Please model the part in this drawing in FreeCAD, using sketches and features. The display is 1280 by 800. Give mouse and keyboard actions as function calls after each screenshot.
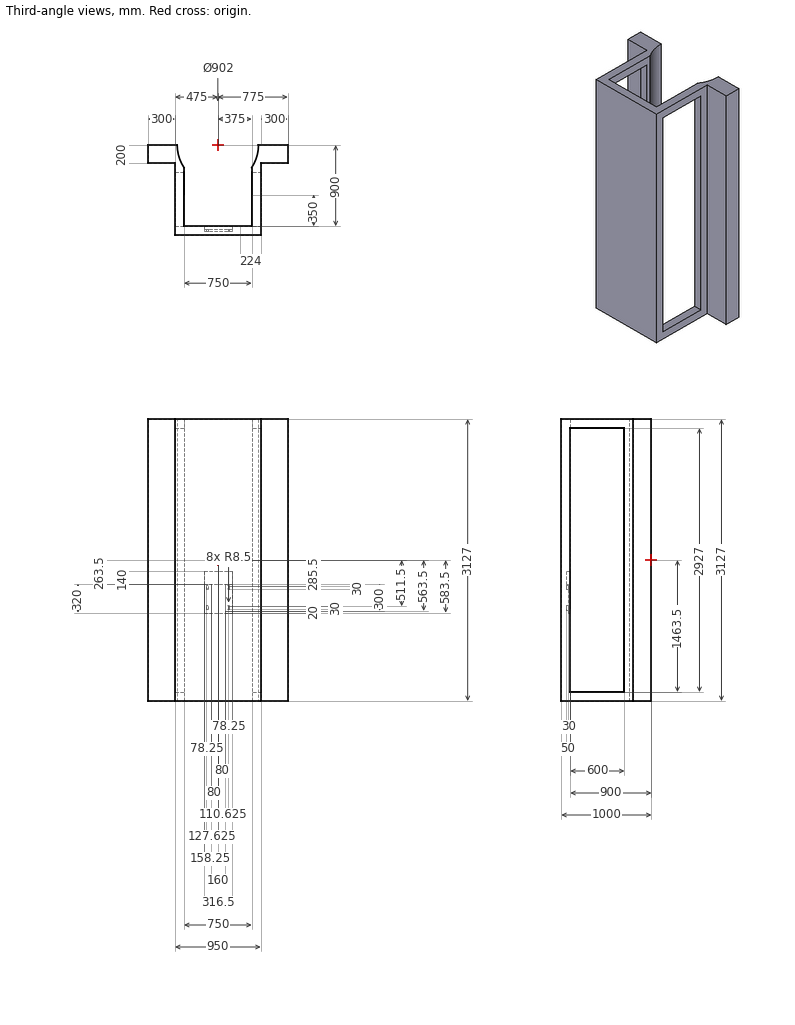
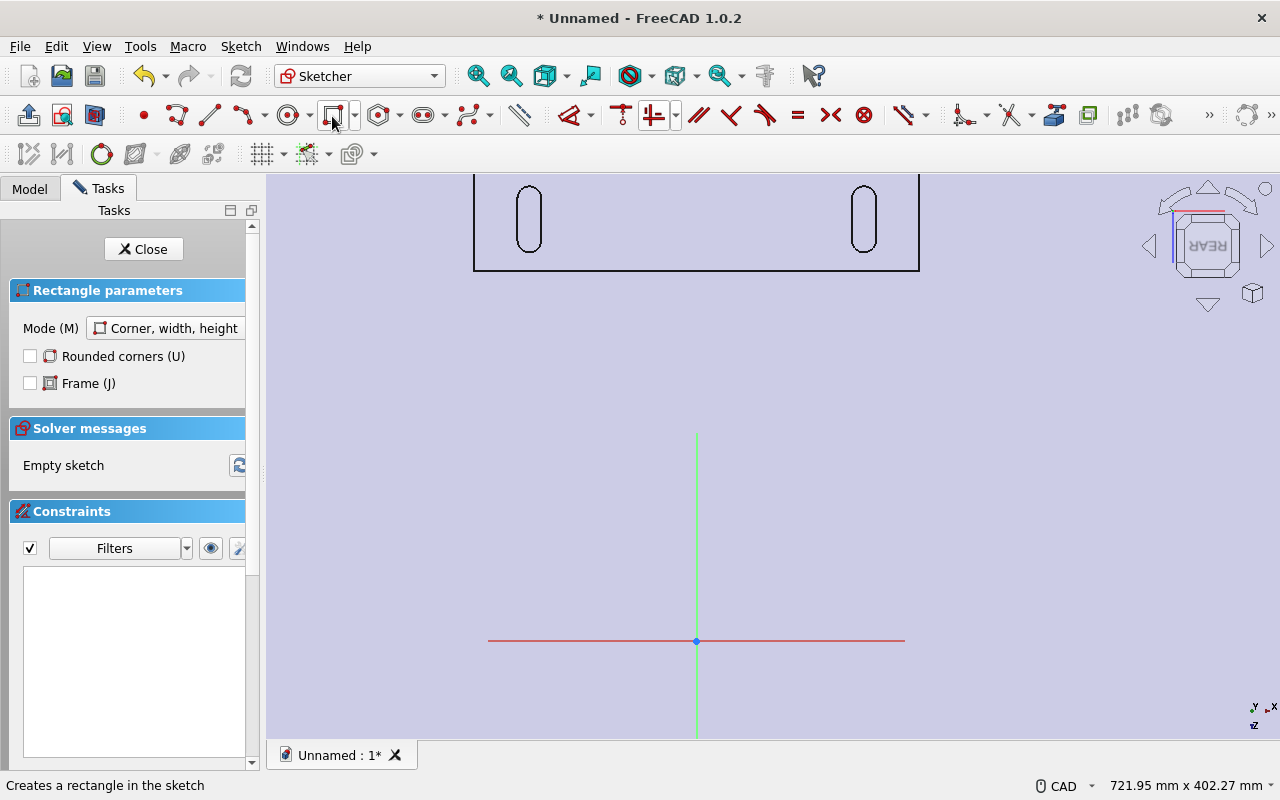
click(474, 271)
click(919, 468)
key(Escape)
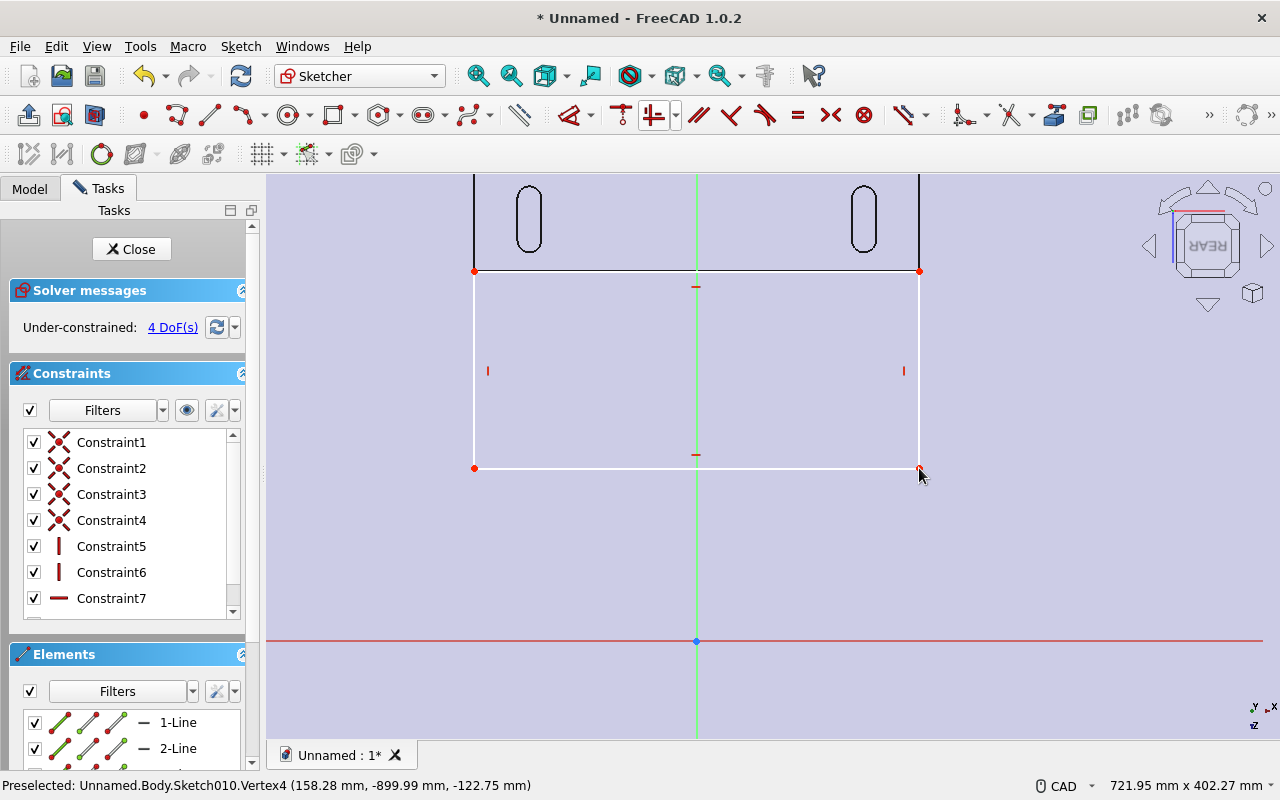
click(568, 116)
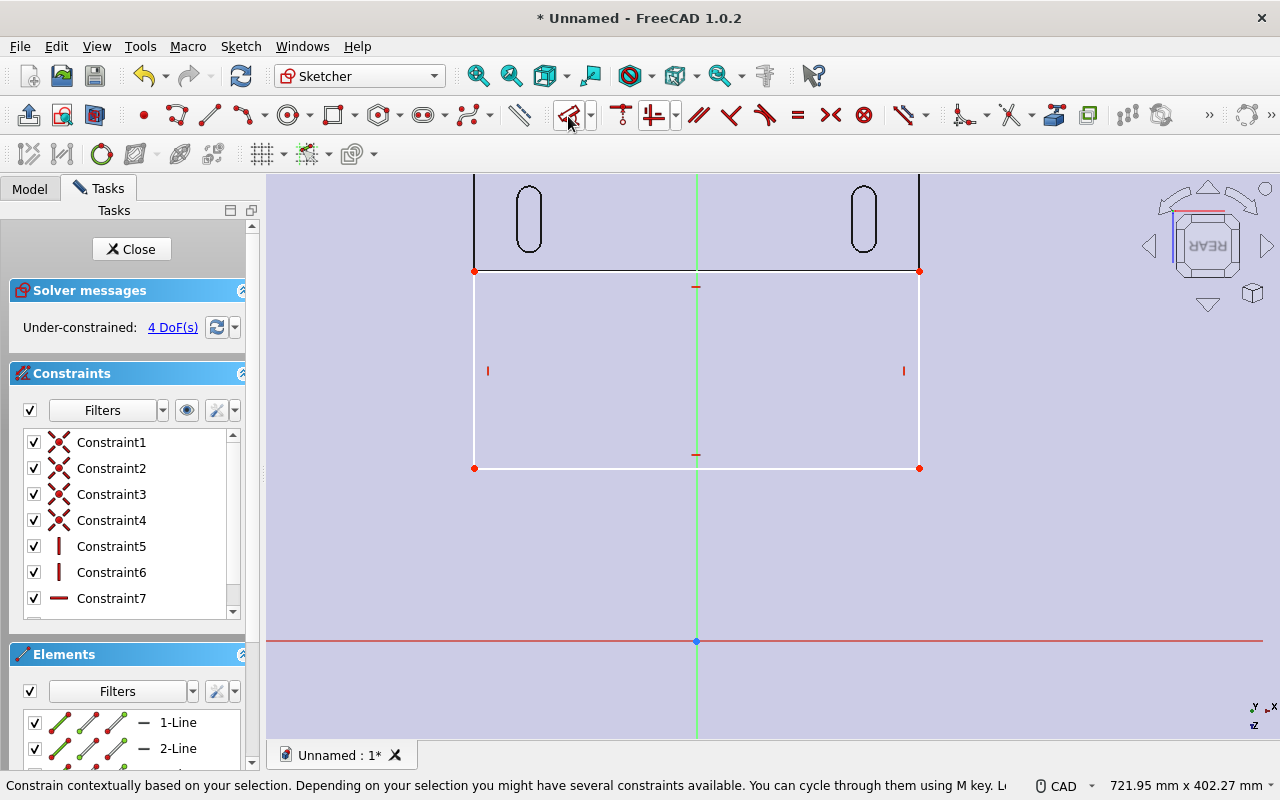
click(474, 331)
click(440, 370)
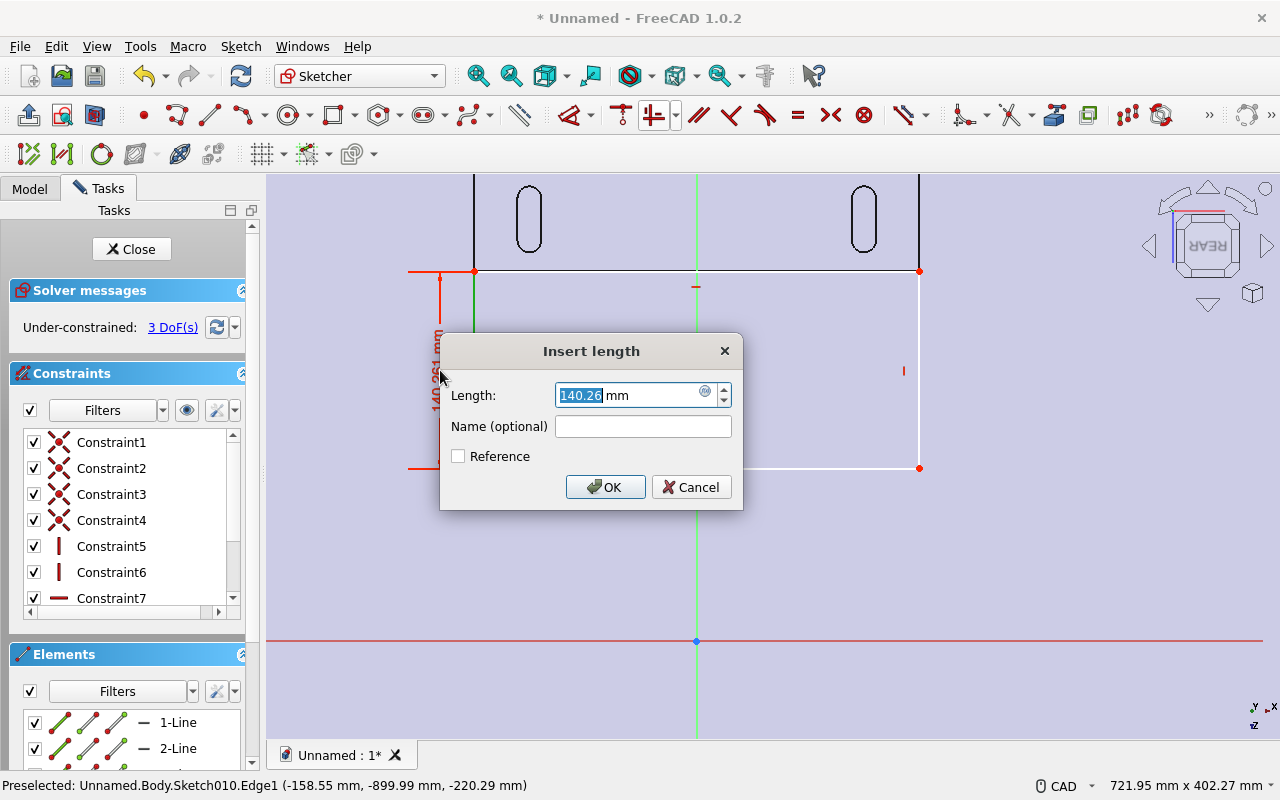
text(140)
key(Return)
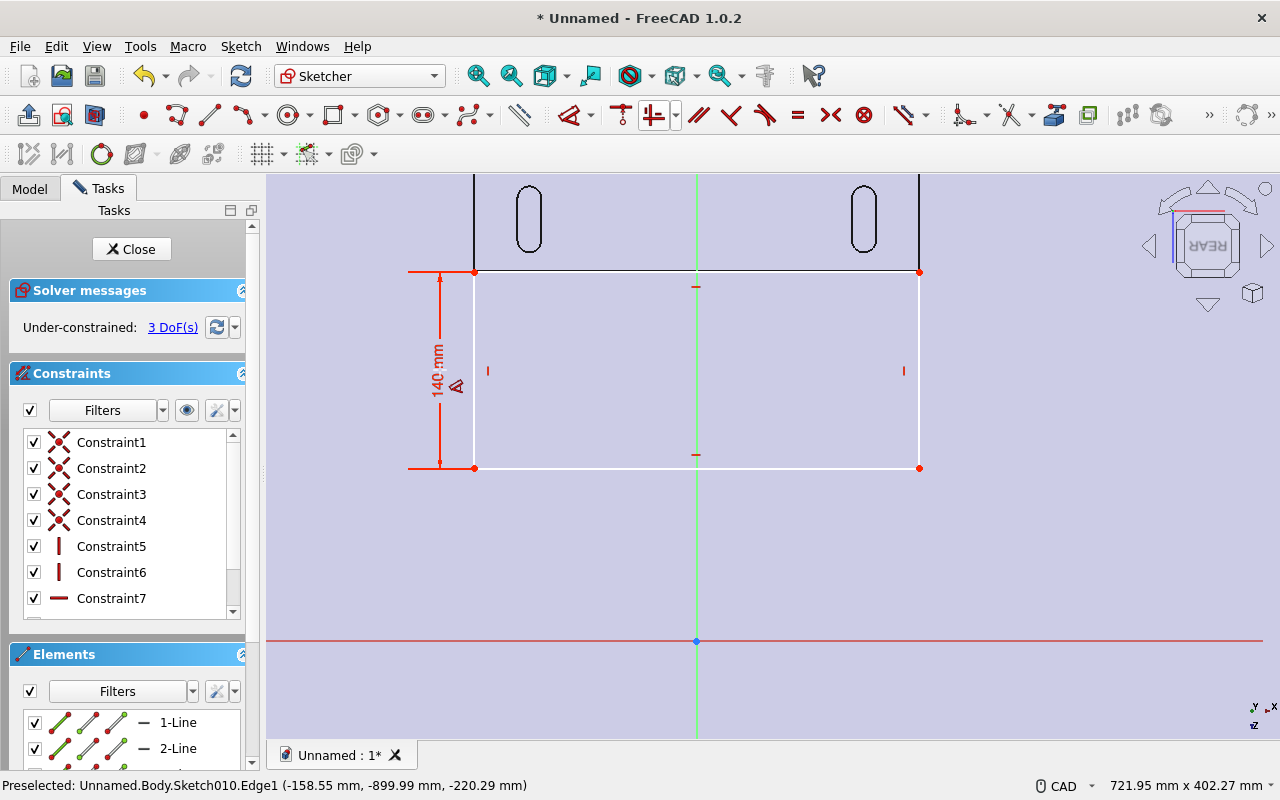
click(607, 469)
click(594, 503)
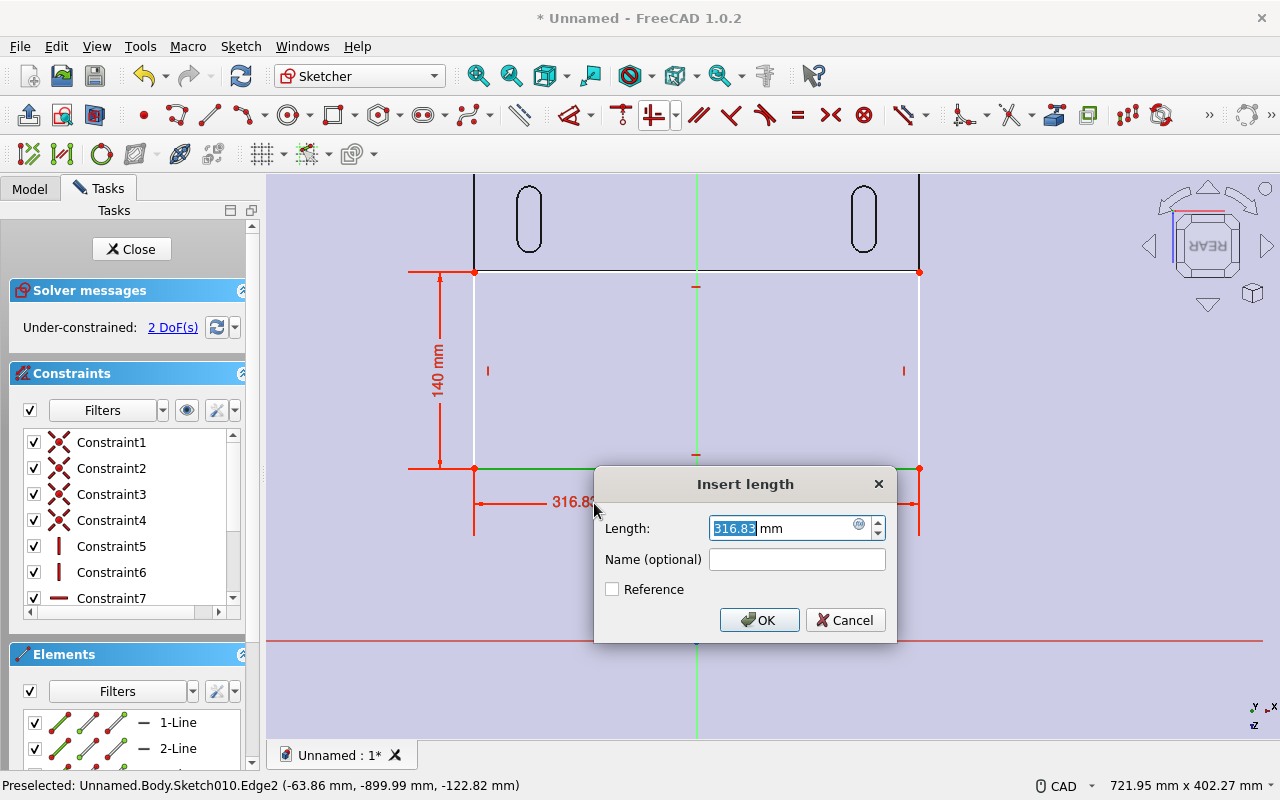
text(316.5)
key(Return)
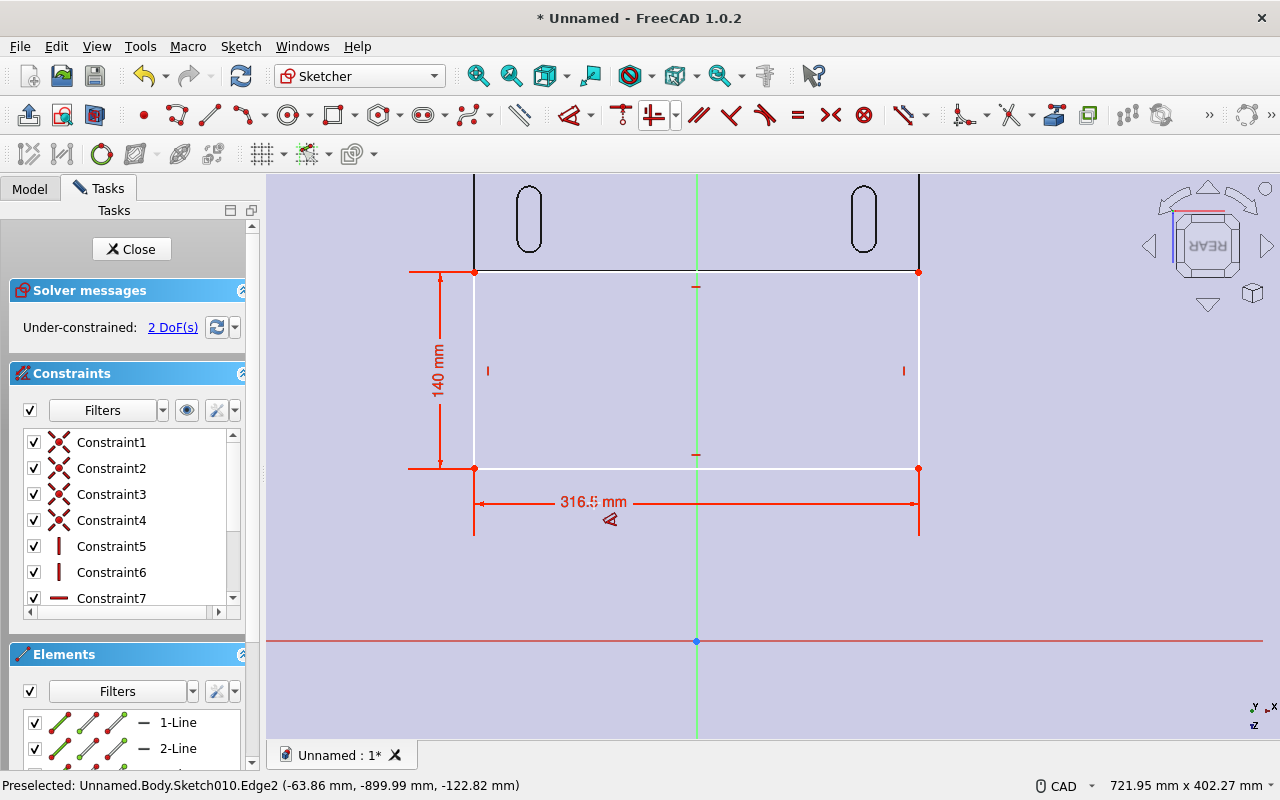
click(474, 272)
click(440, 457)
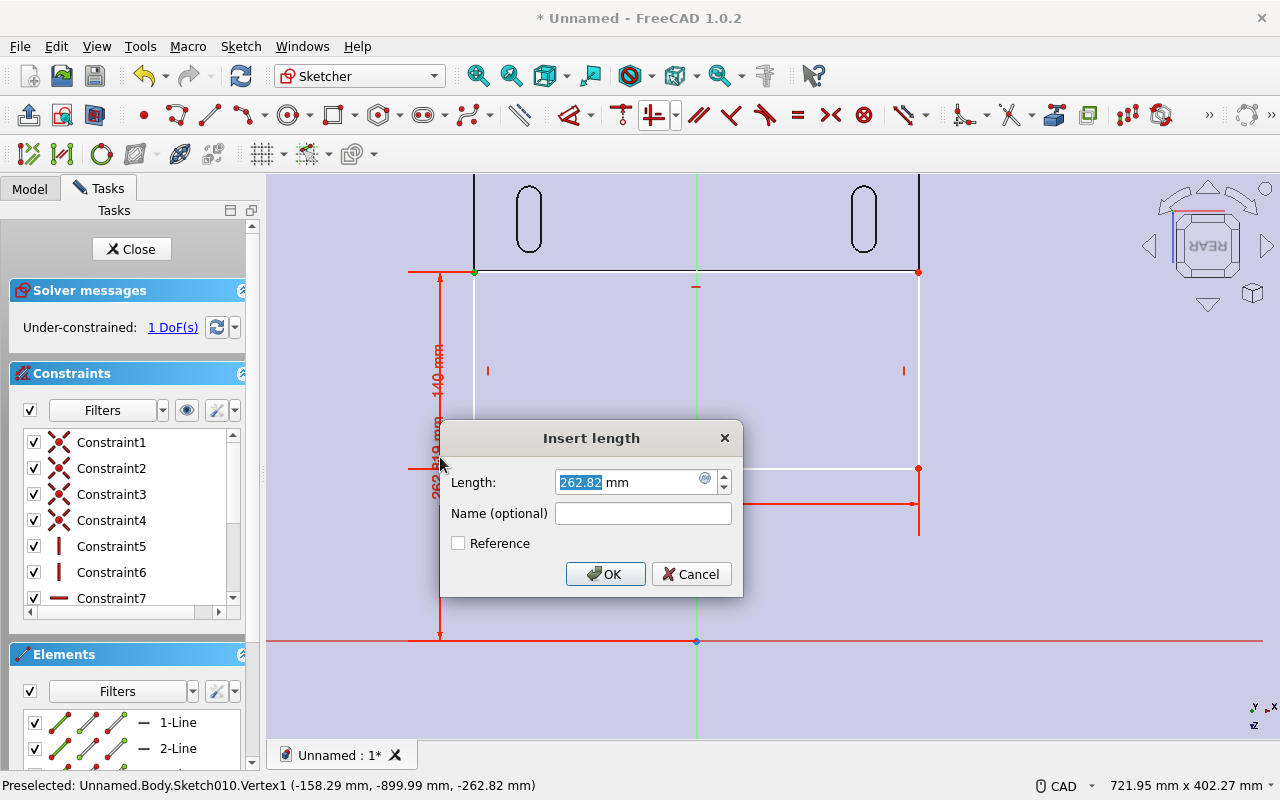
text(263.5)
key(Return)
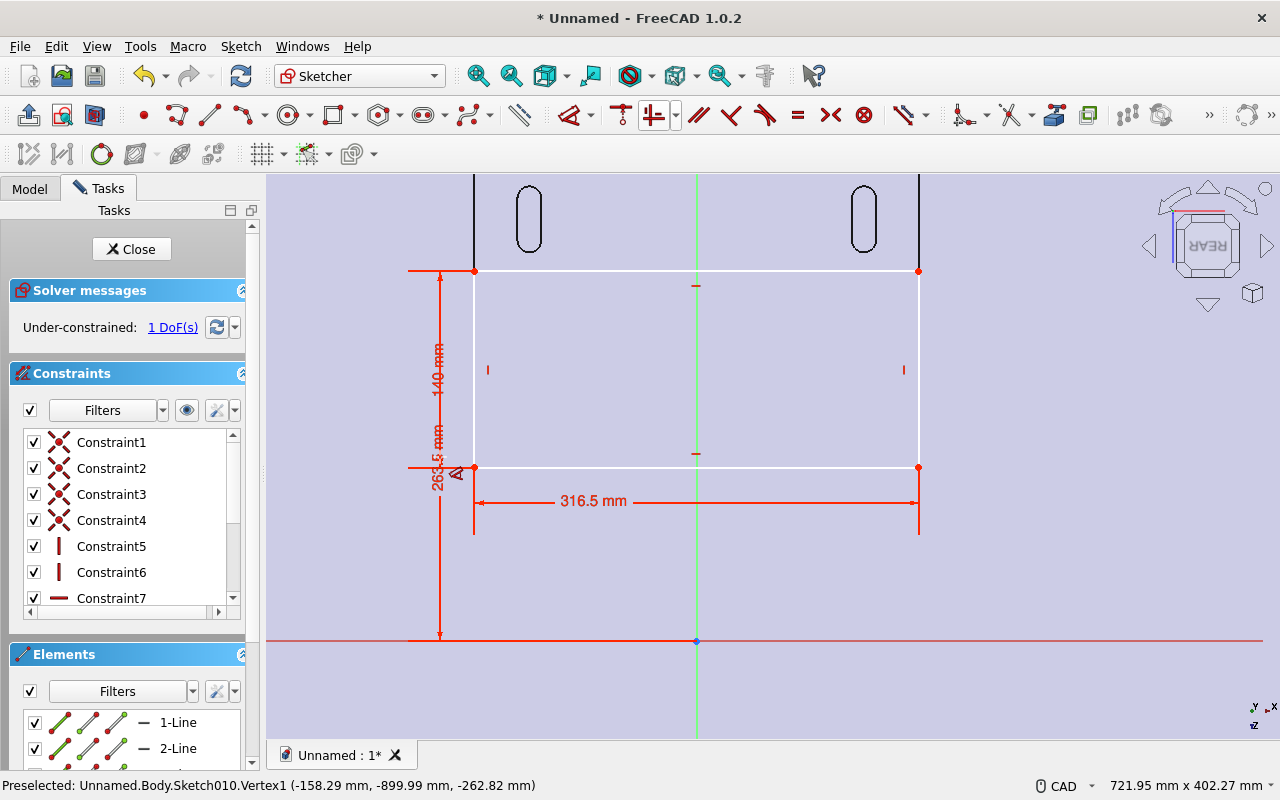
click(474, 271)
click(586, 675)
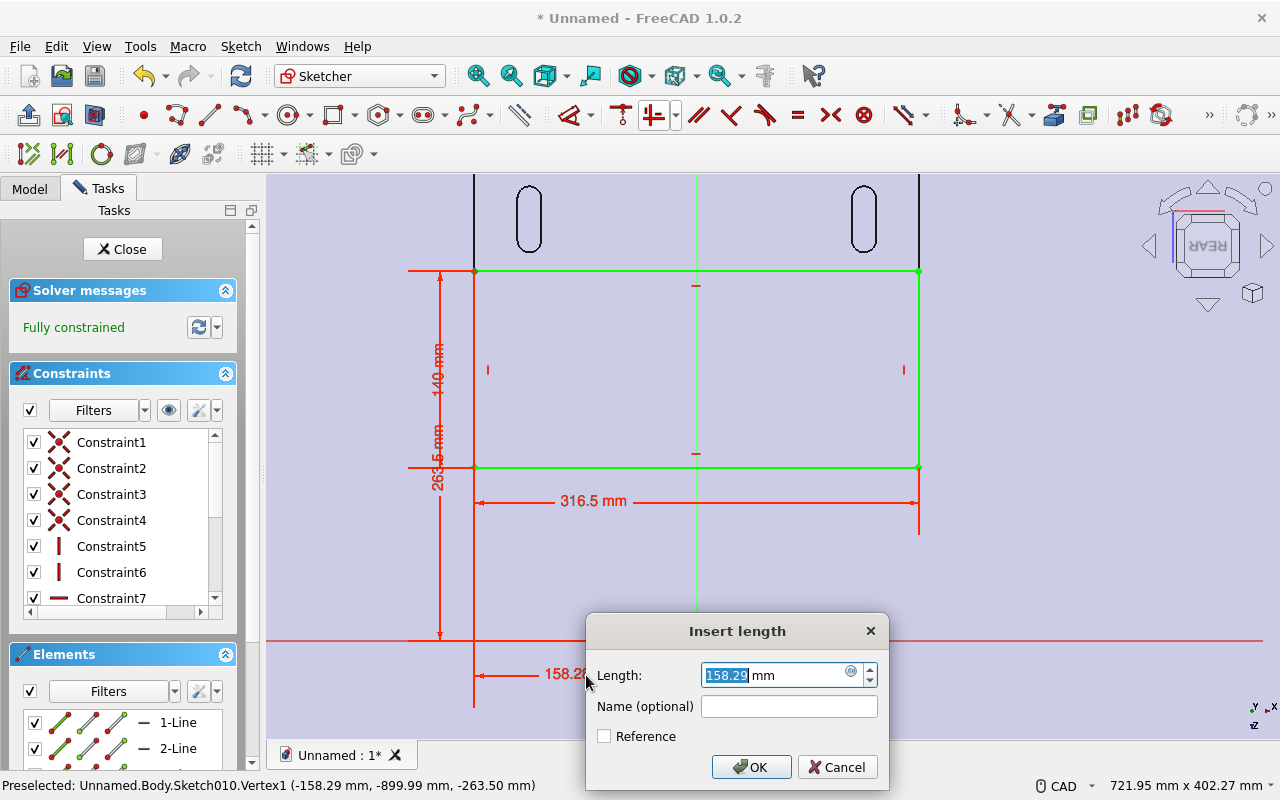
text(158.25)
key(Return)
key(Escape)